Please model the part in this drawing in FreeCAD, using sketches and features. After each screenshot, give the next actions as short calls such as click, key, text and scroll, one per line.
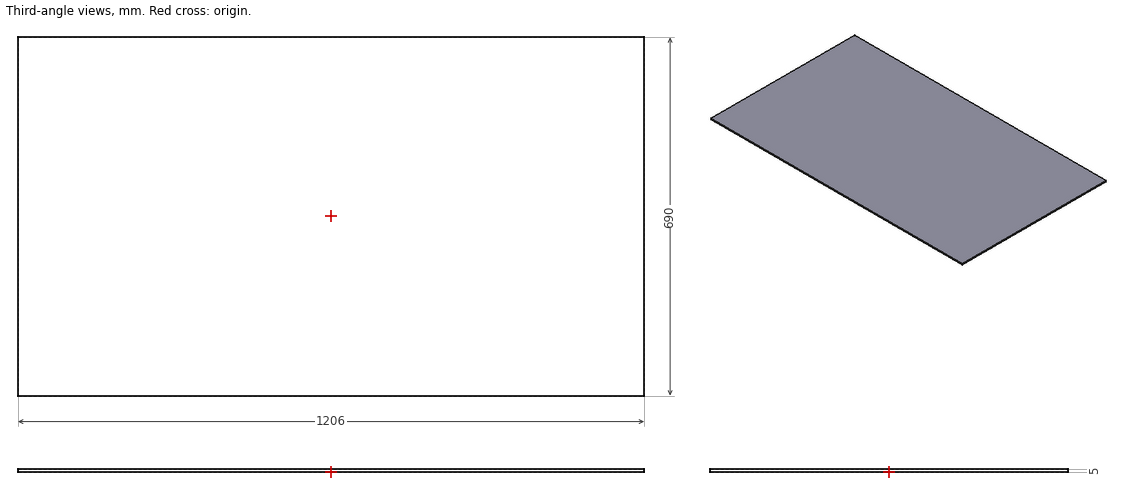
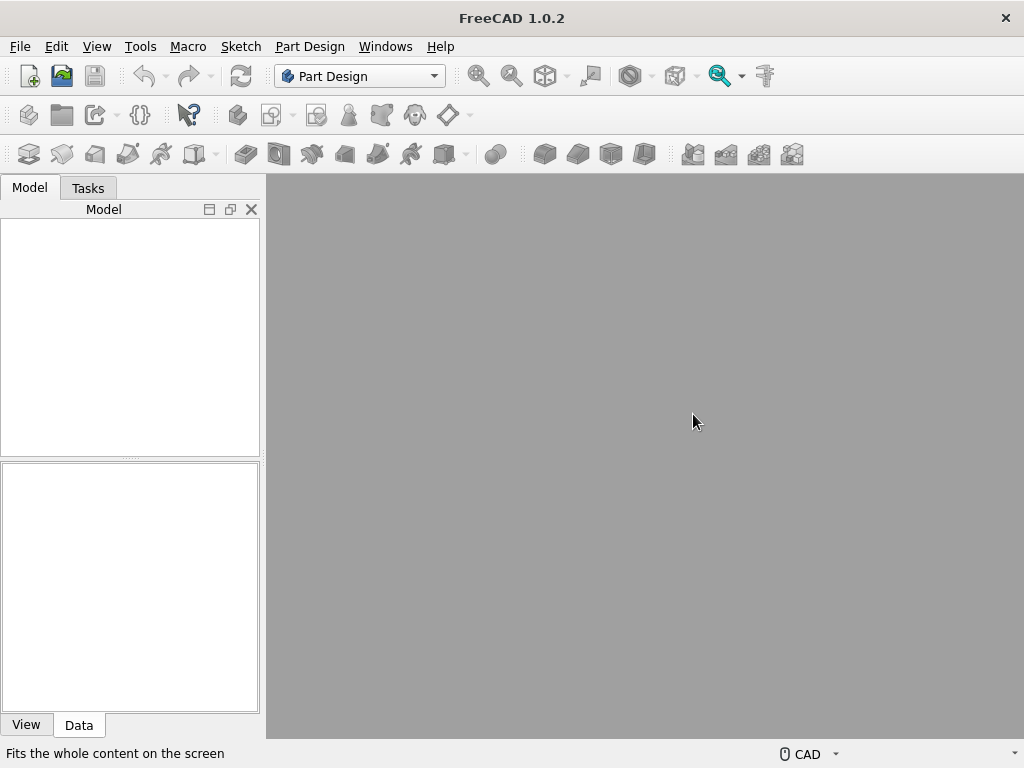
key(ctrl+n)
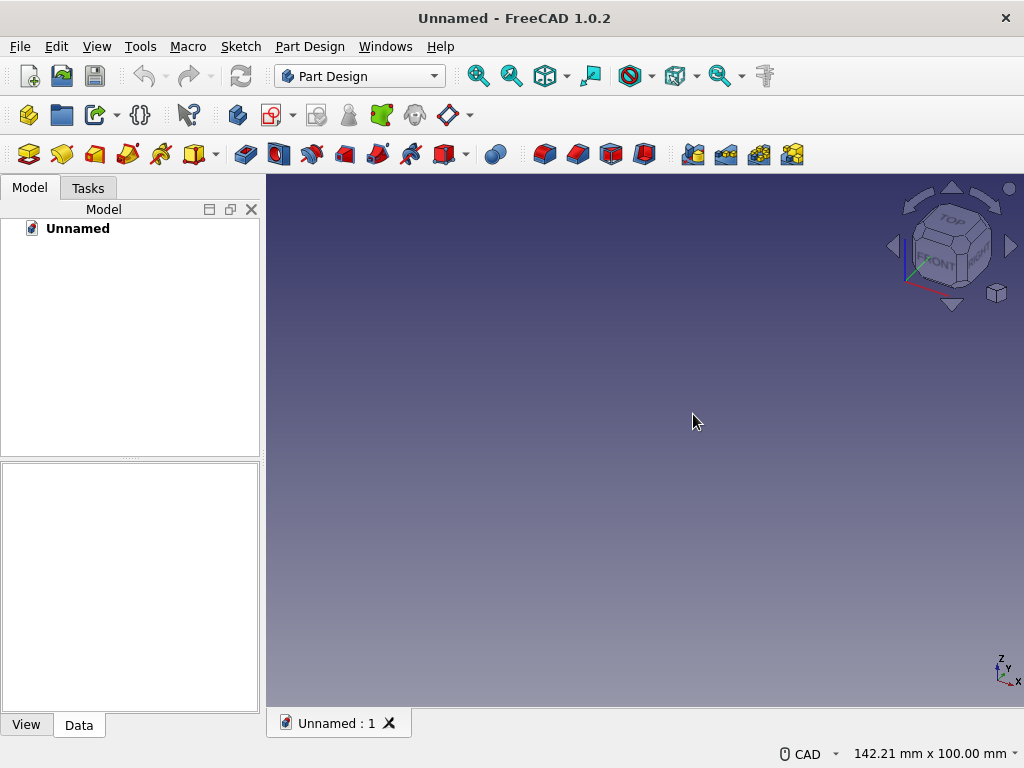
click(270, 116)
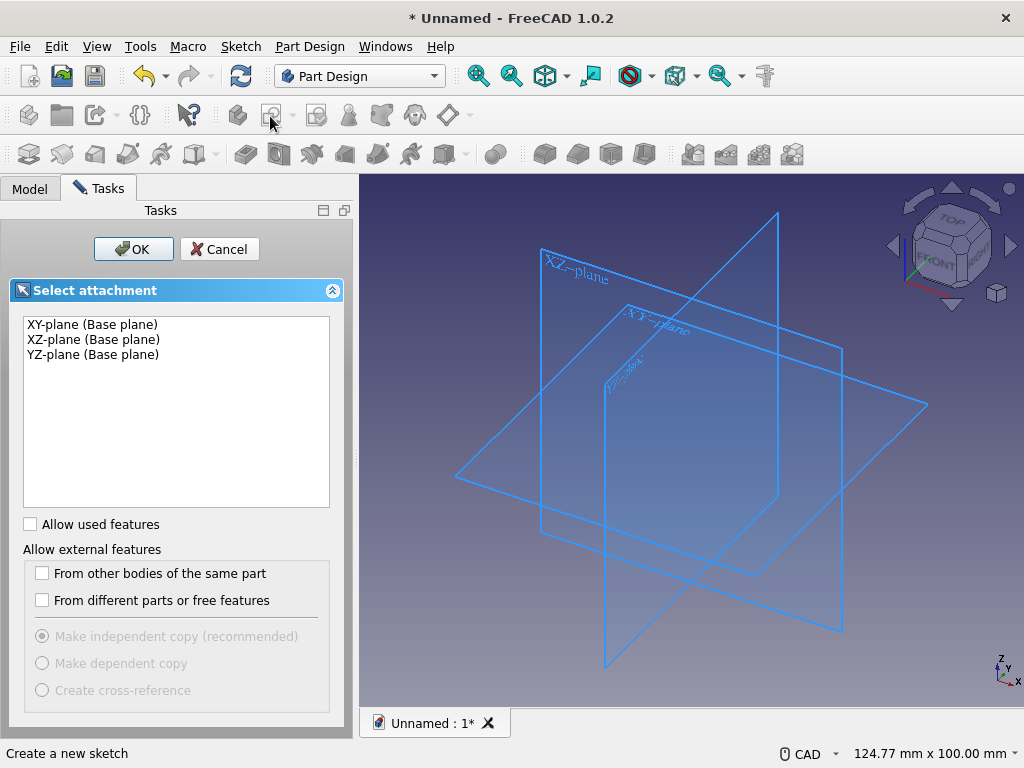
click(84, 324)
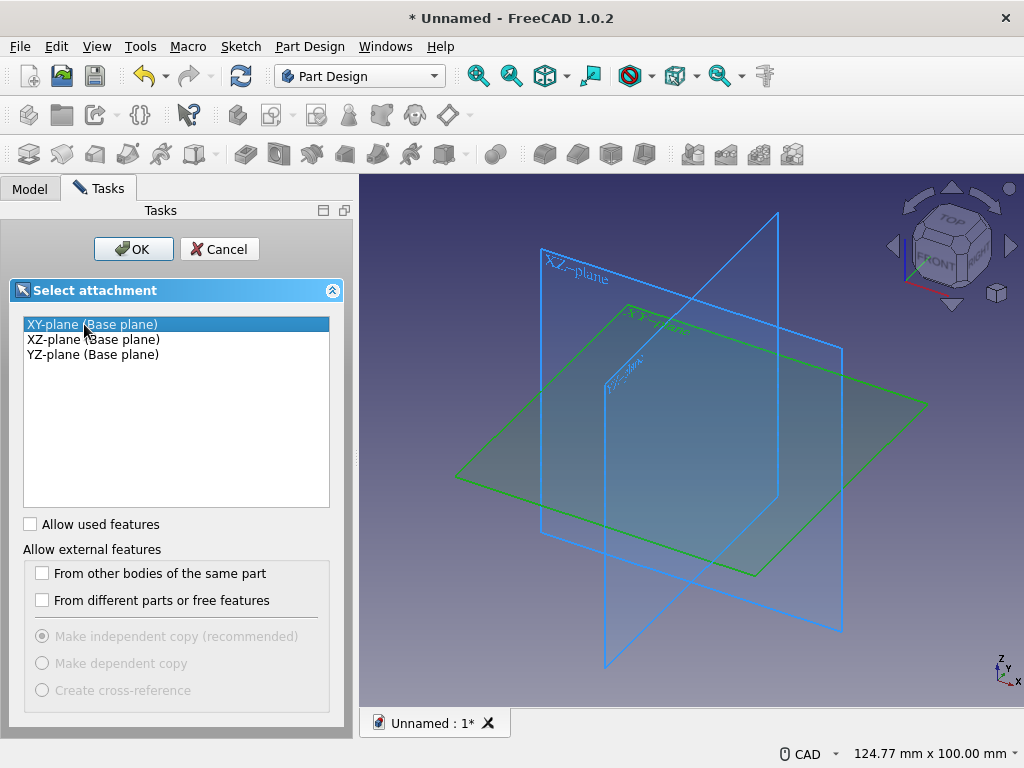
click(134, 249)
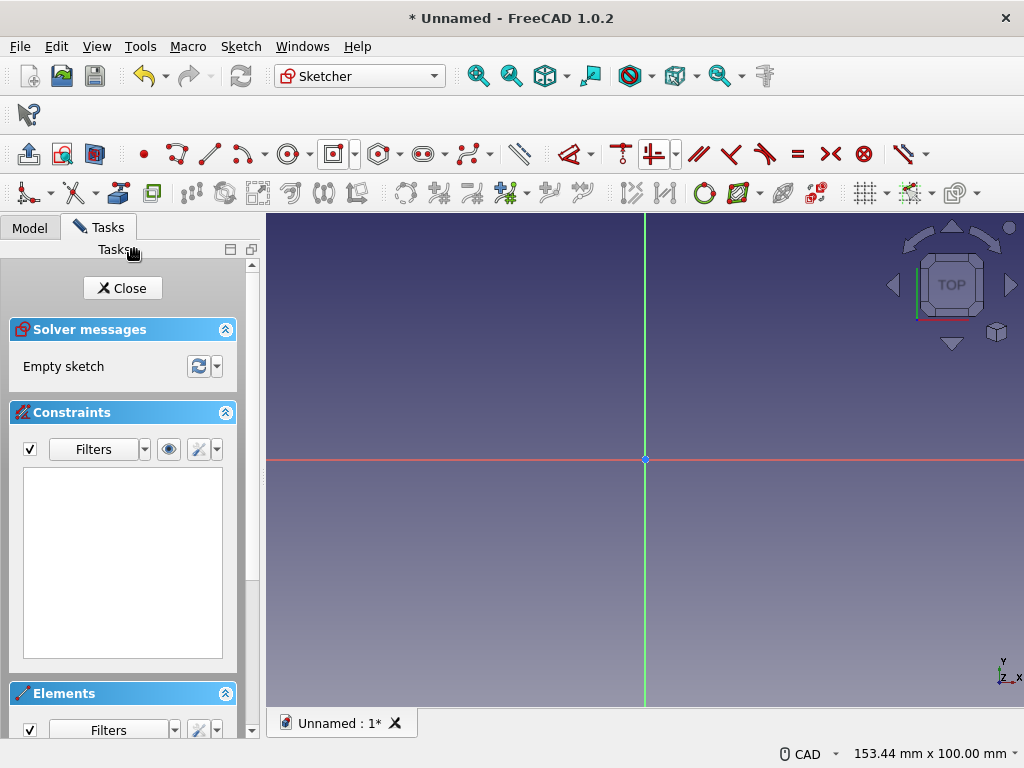
scroll(572, 460, down, 14)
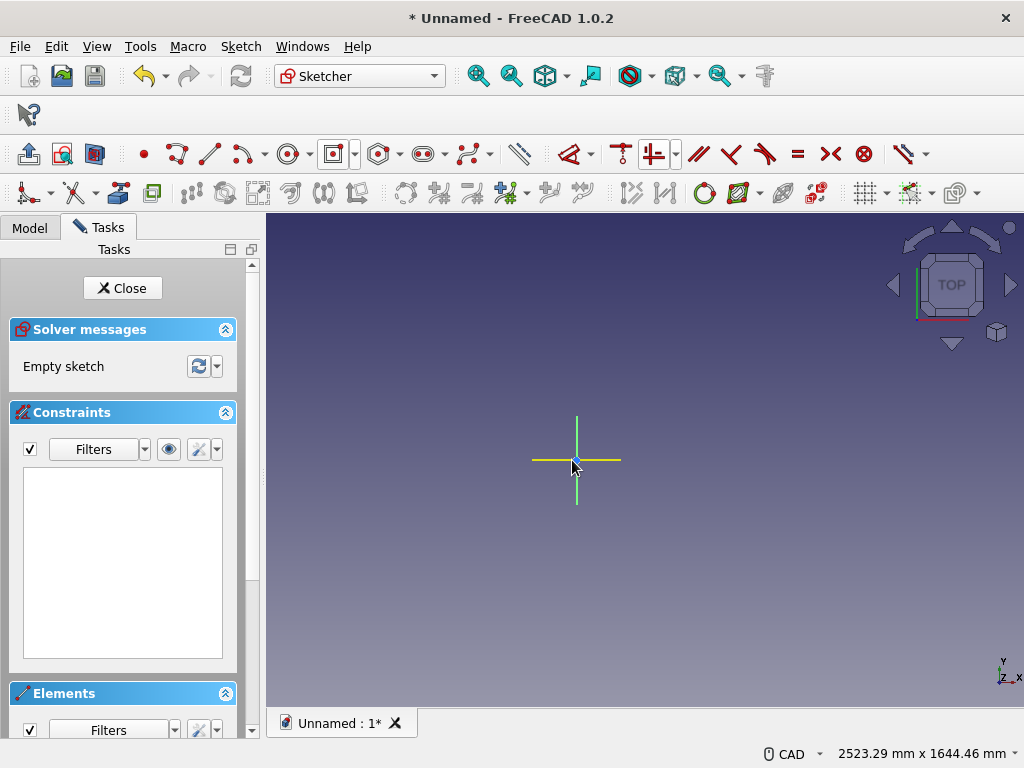
key(g)
key(v)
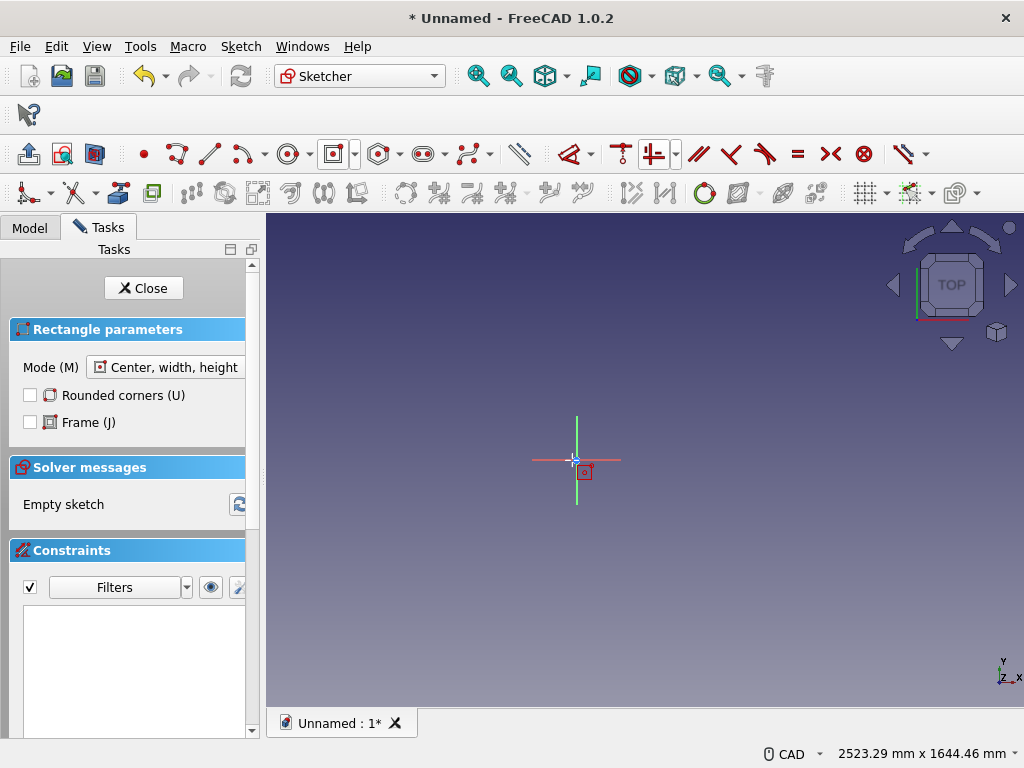
click(577, 460)
move(758, 357)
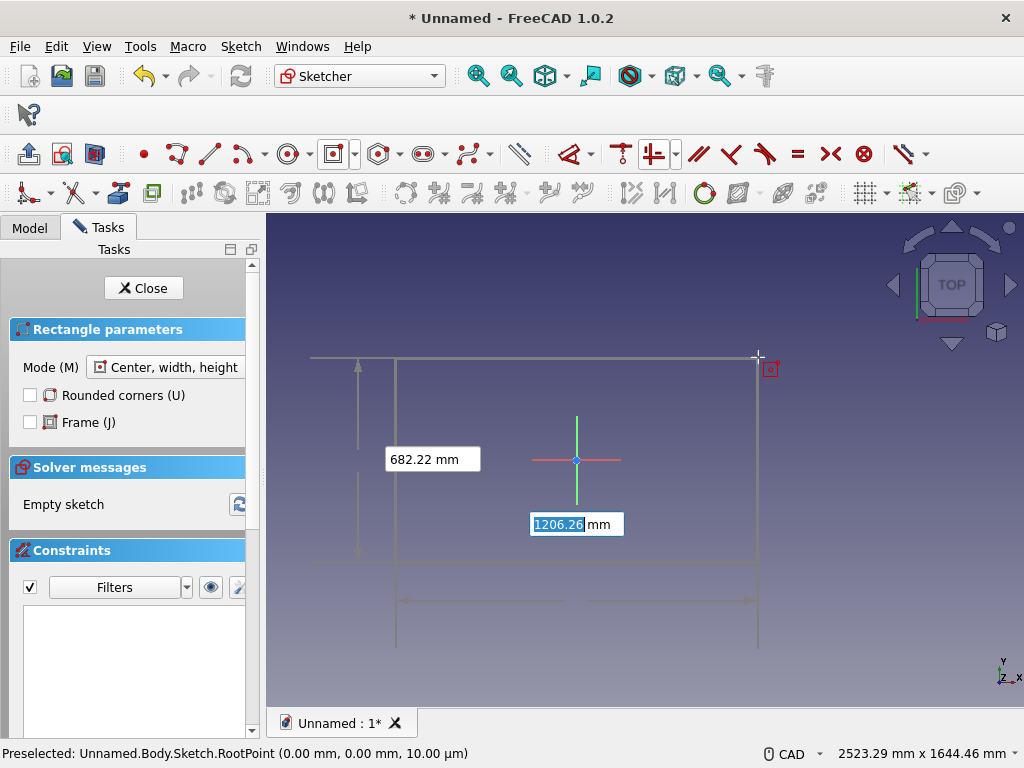
text(1206)
key(Tab)
text(690)
key(Return)
key(Escape)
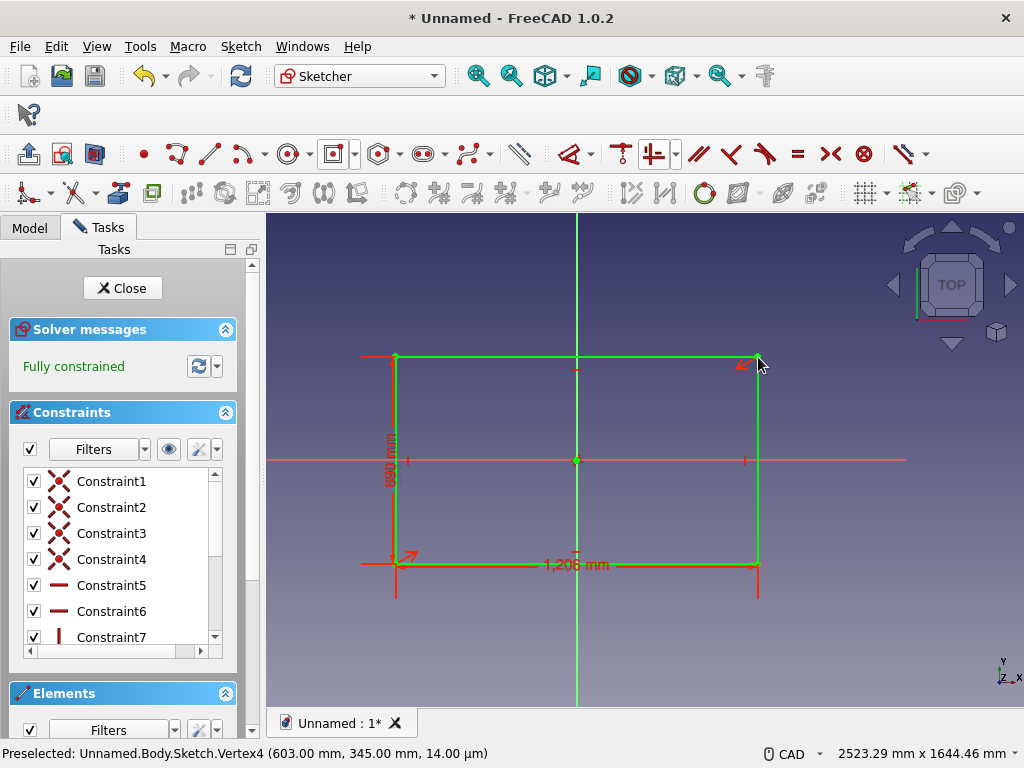
click(123, 288)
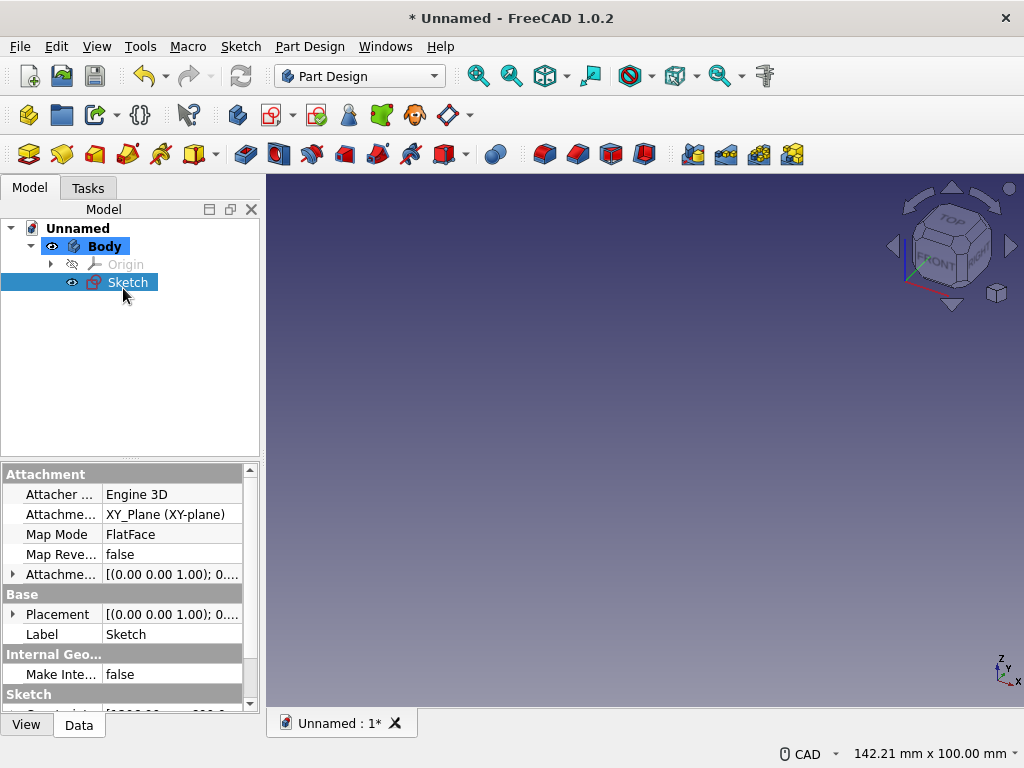
click(29, 154)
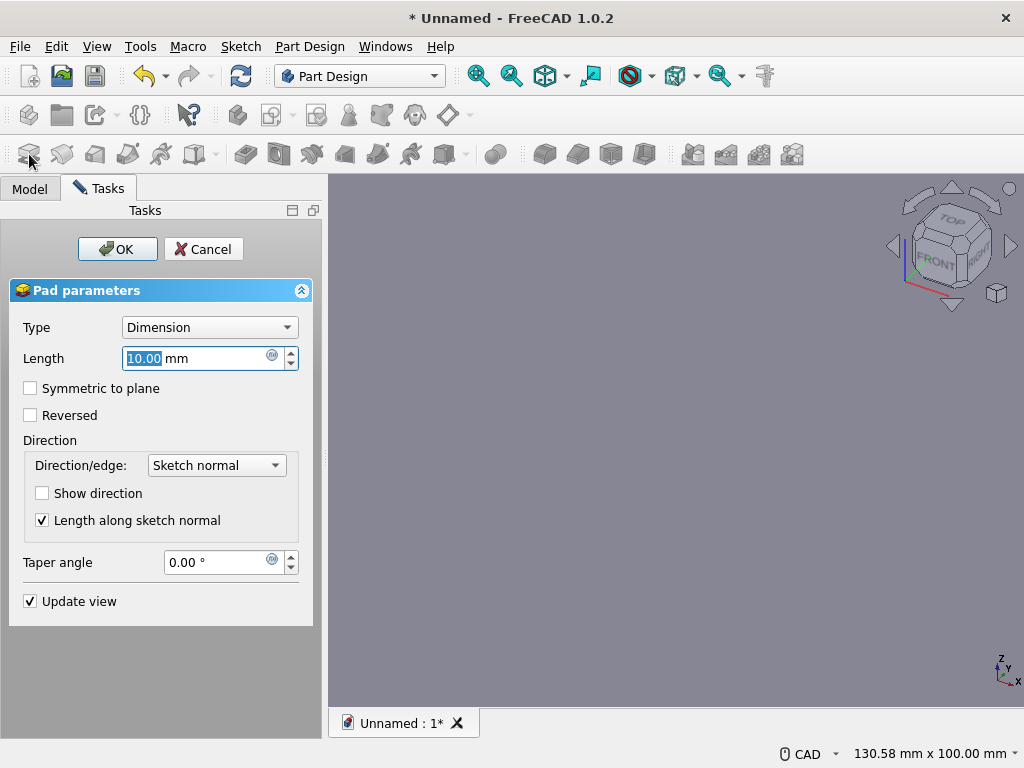
text(5)
key(Tab)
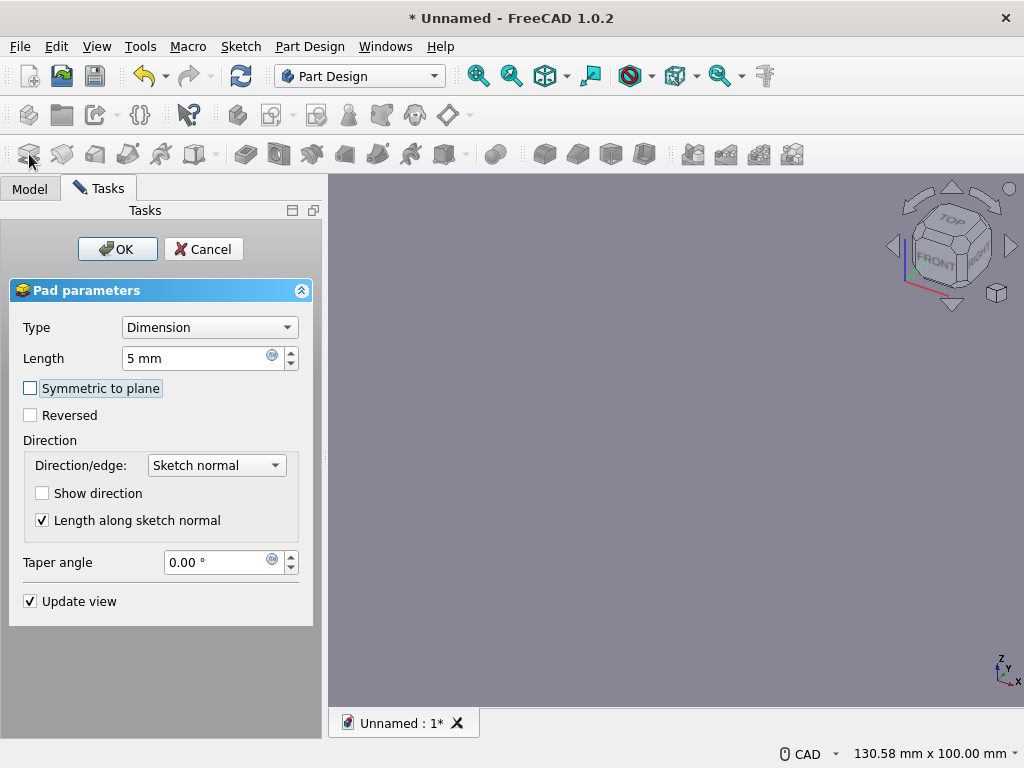
click(118, 249)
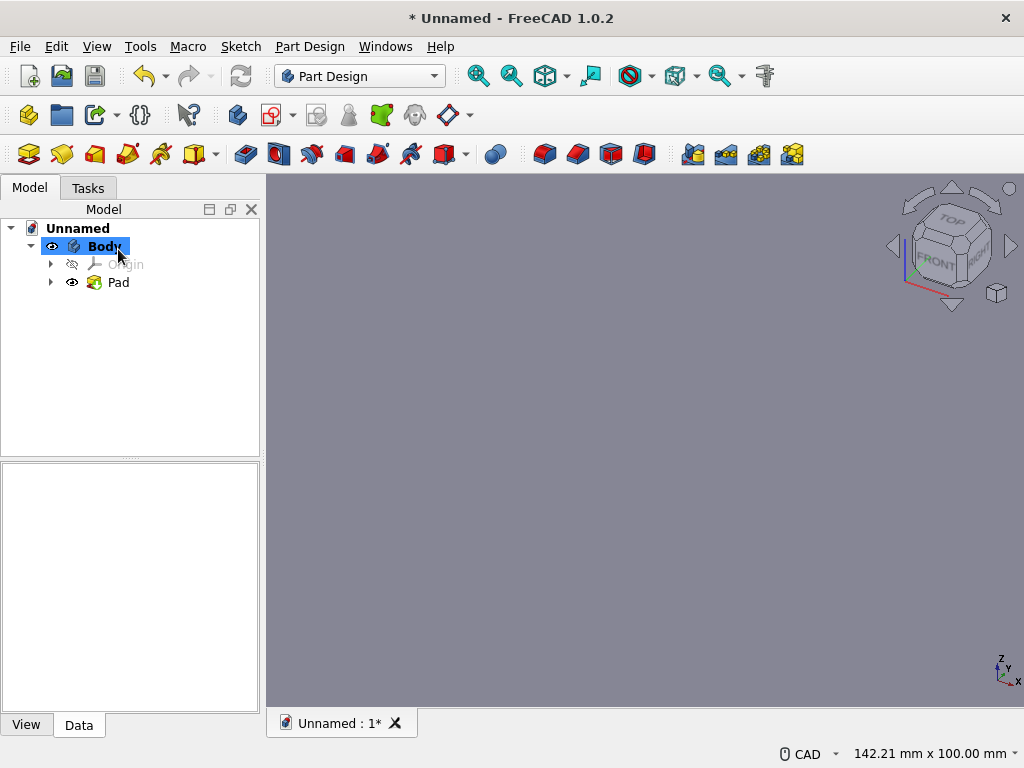
key(0)